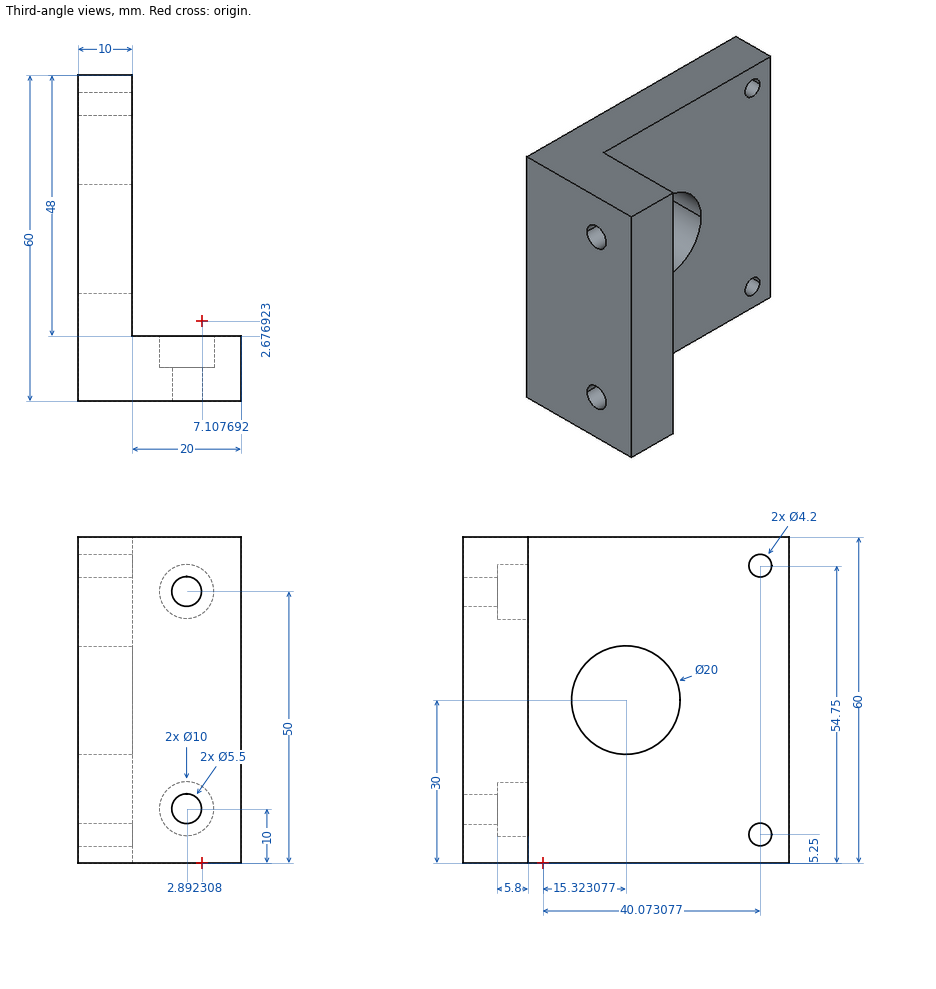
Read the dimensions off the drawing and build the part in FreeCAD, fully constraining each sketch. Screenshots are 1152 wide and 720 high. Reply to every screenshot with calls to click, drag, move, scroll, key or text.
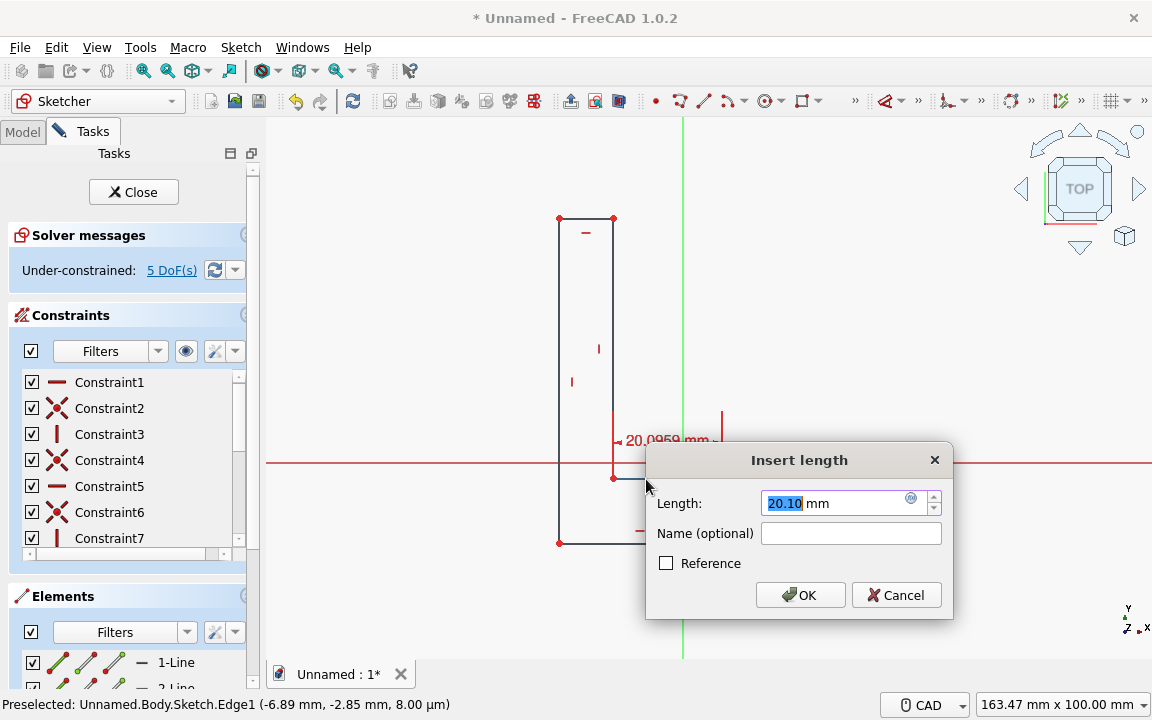
text(20)
key(Return)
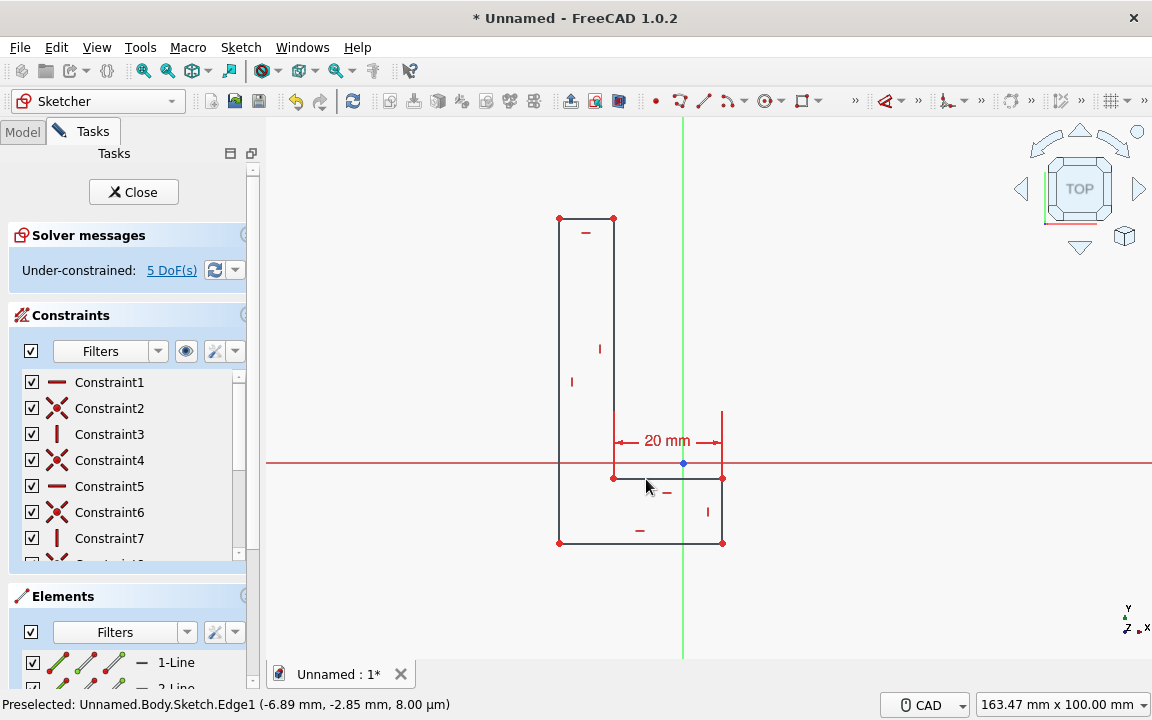
click(614, 401)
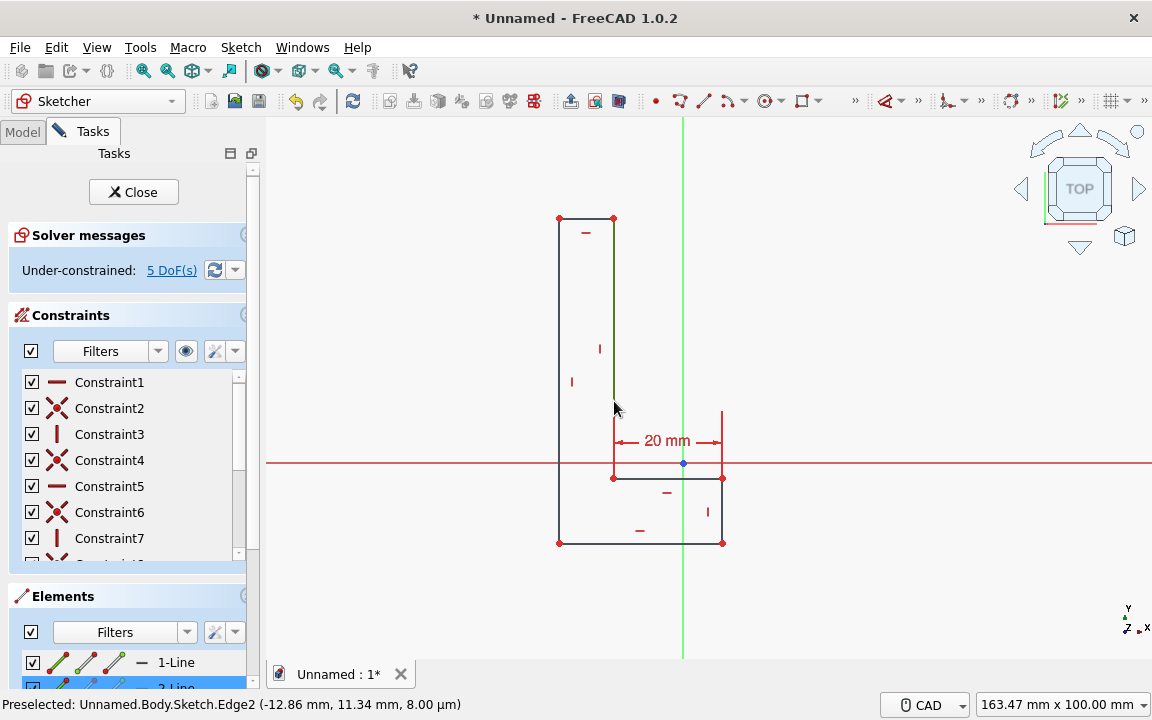
key(i)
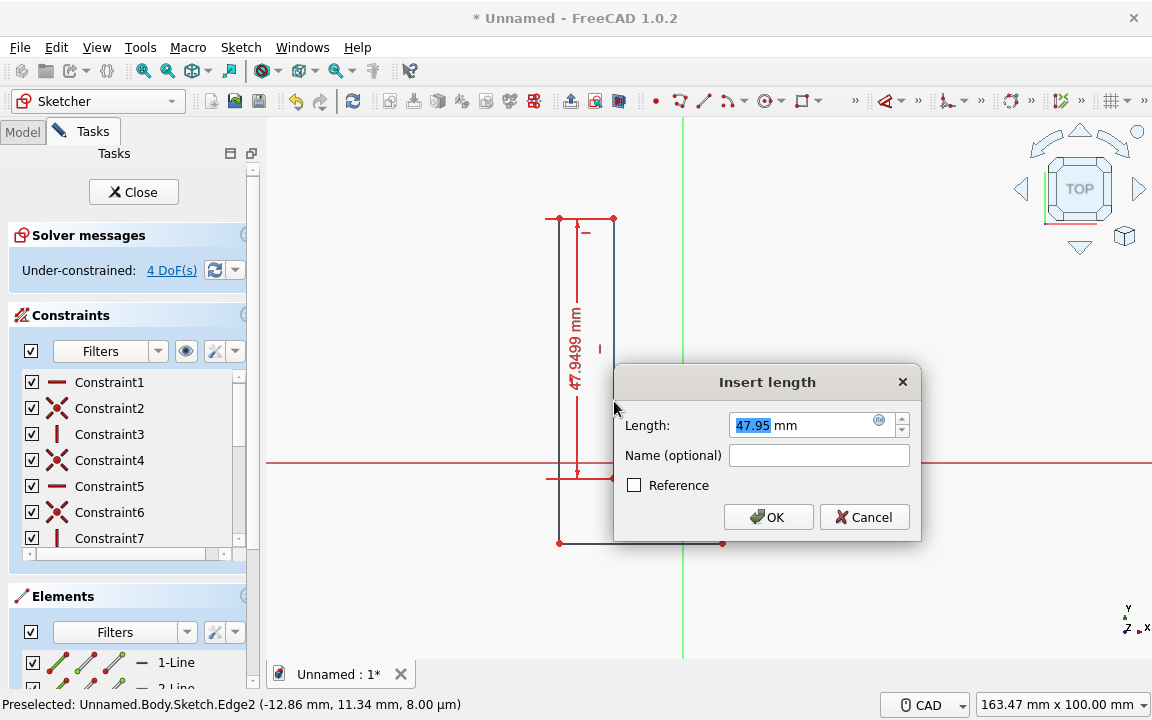
text(48)
key(Return)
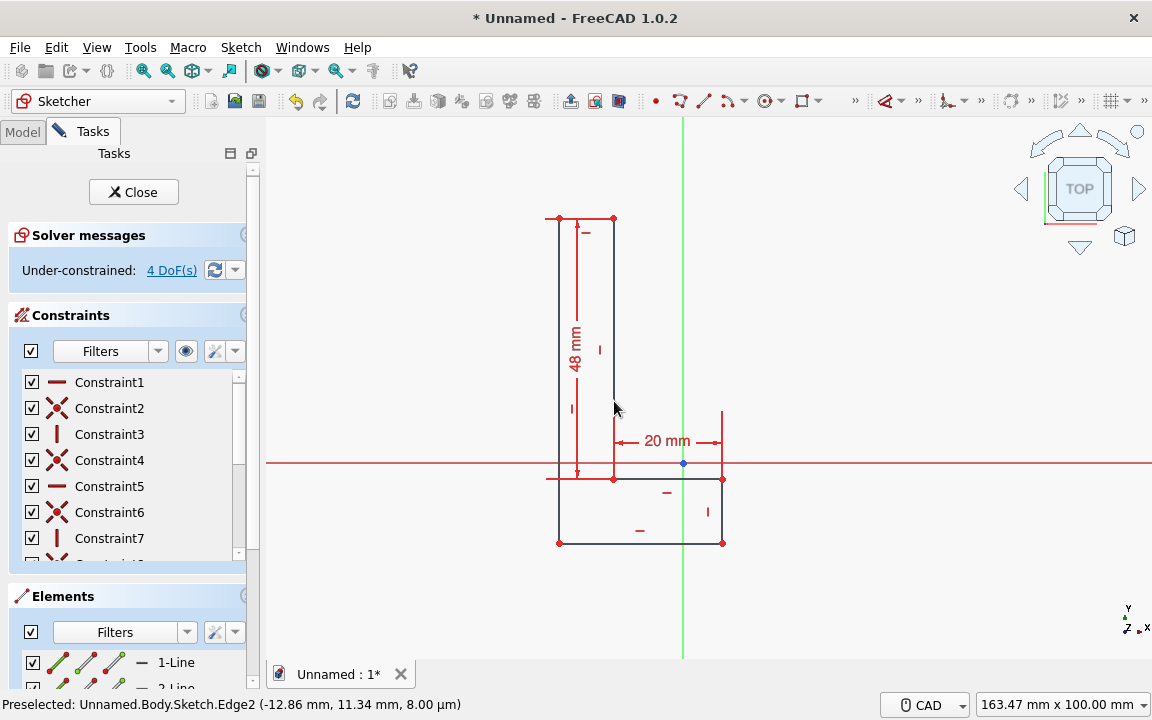
click(597, 219)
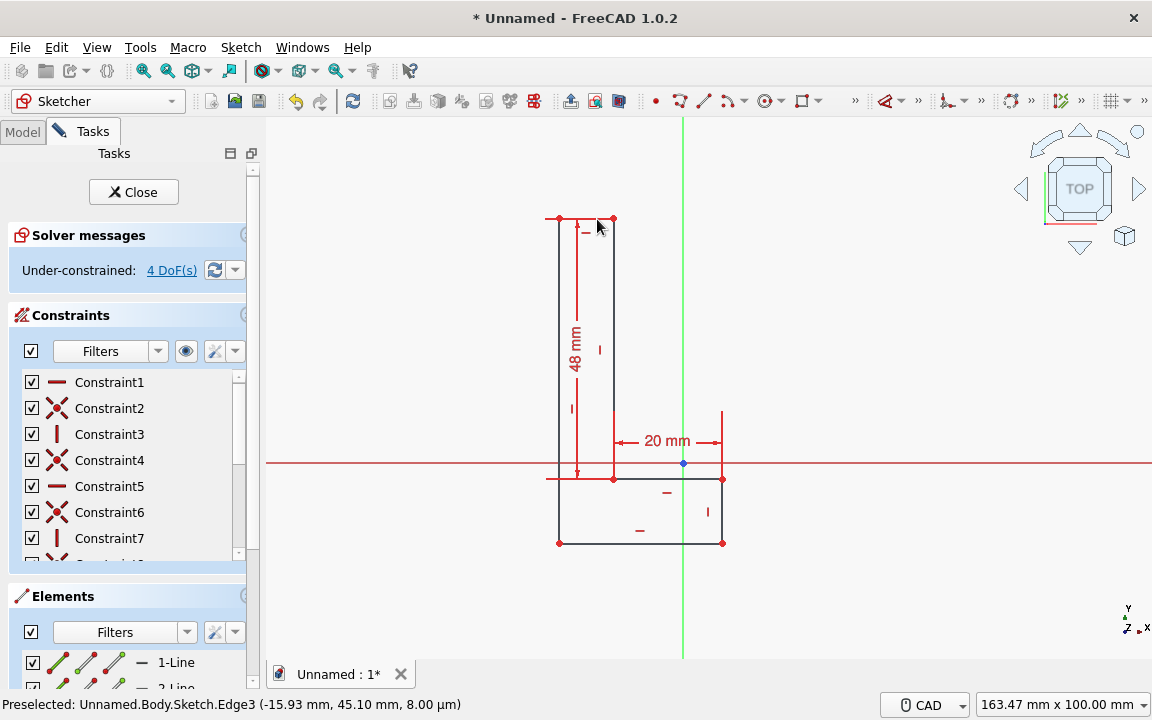
key(l)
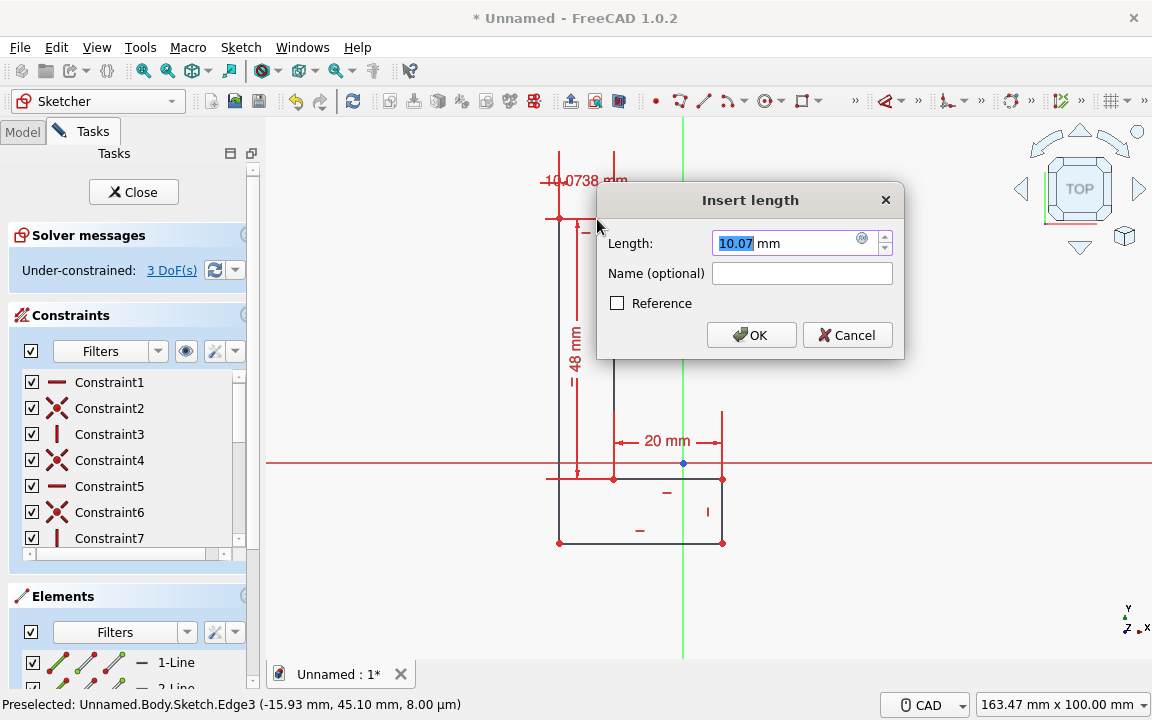
text(10)
key(Return)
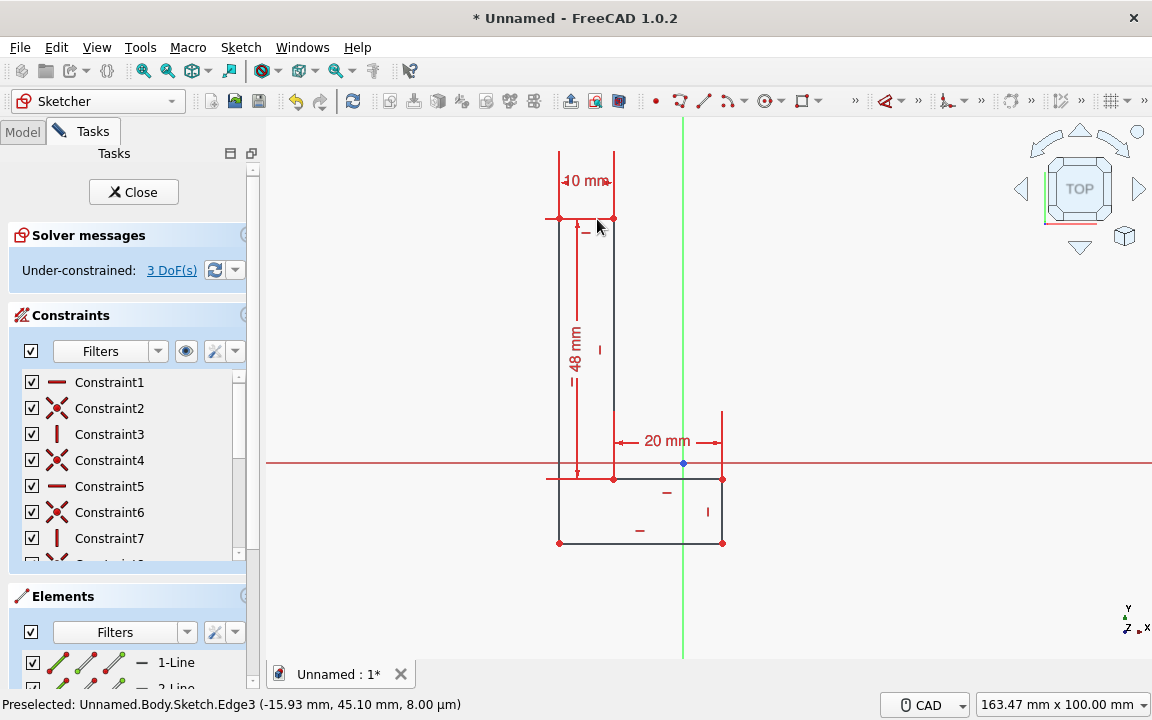
click(559, 317)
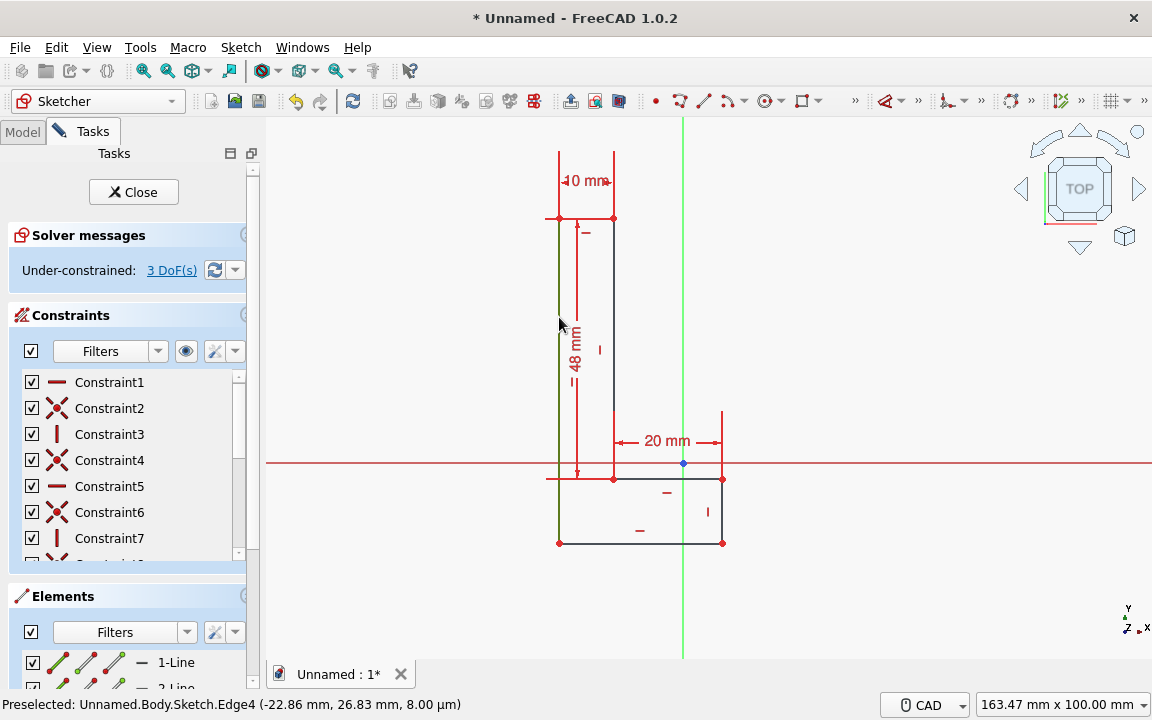
click(904, 102)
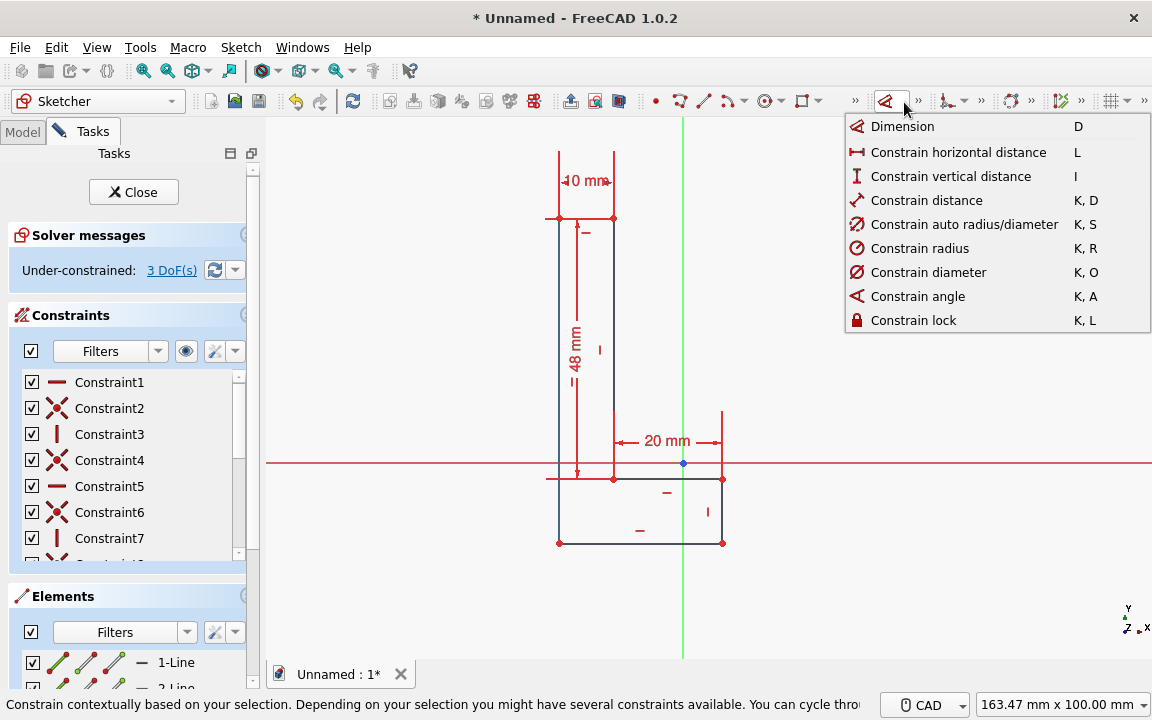
click(998, 176)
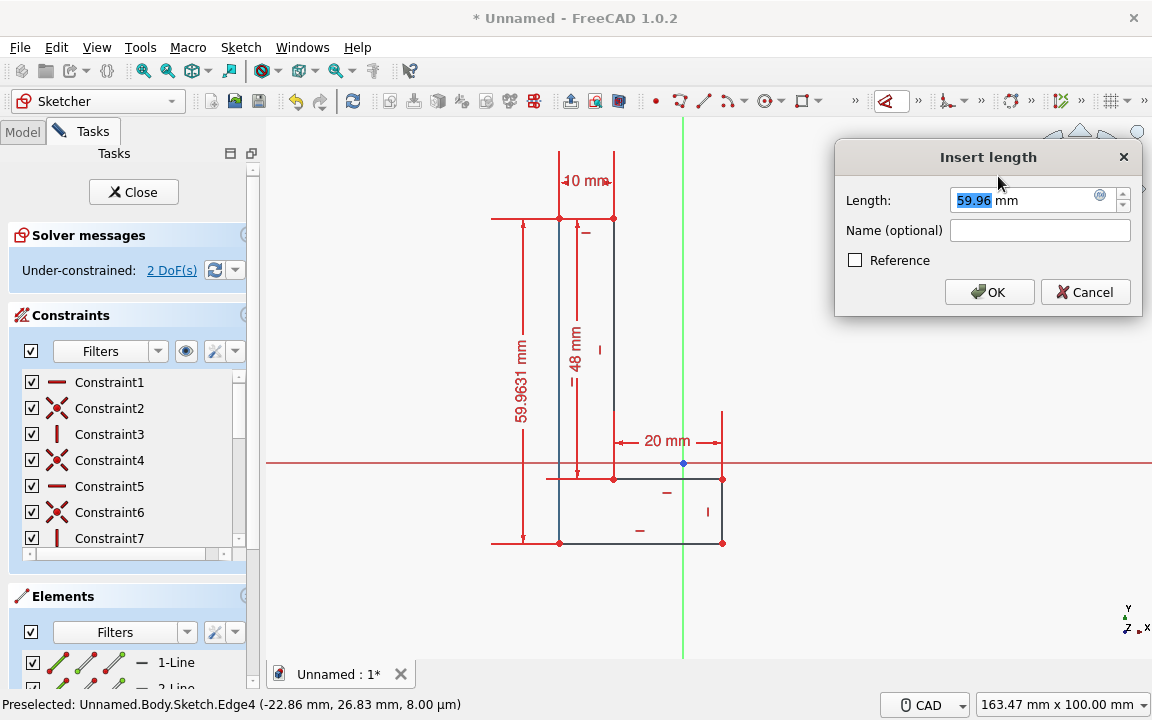
text(60)
key(Return)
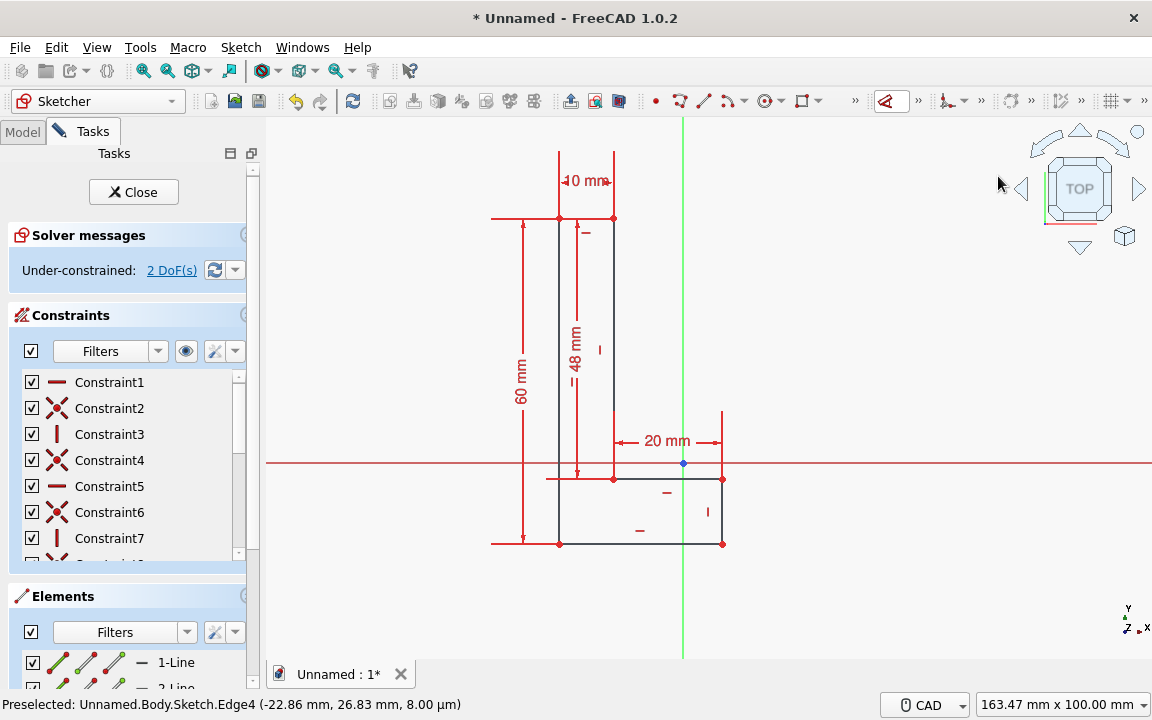
click(722, 479)